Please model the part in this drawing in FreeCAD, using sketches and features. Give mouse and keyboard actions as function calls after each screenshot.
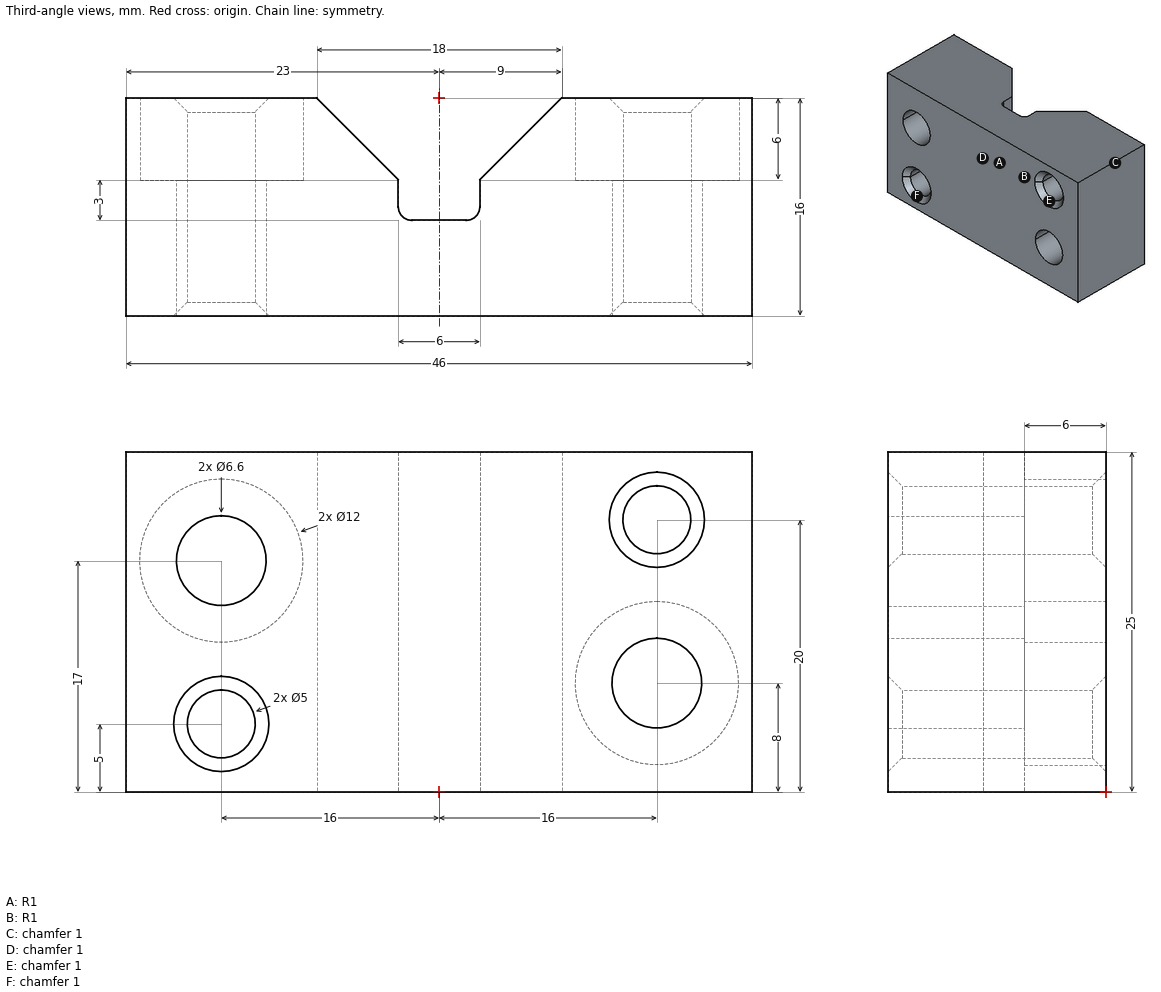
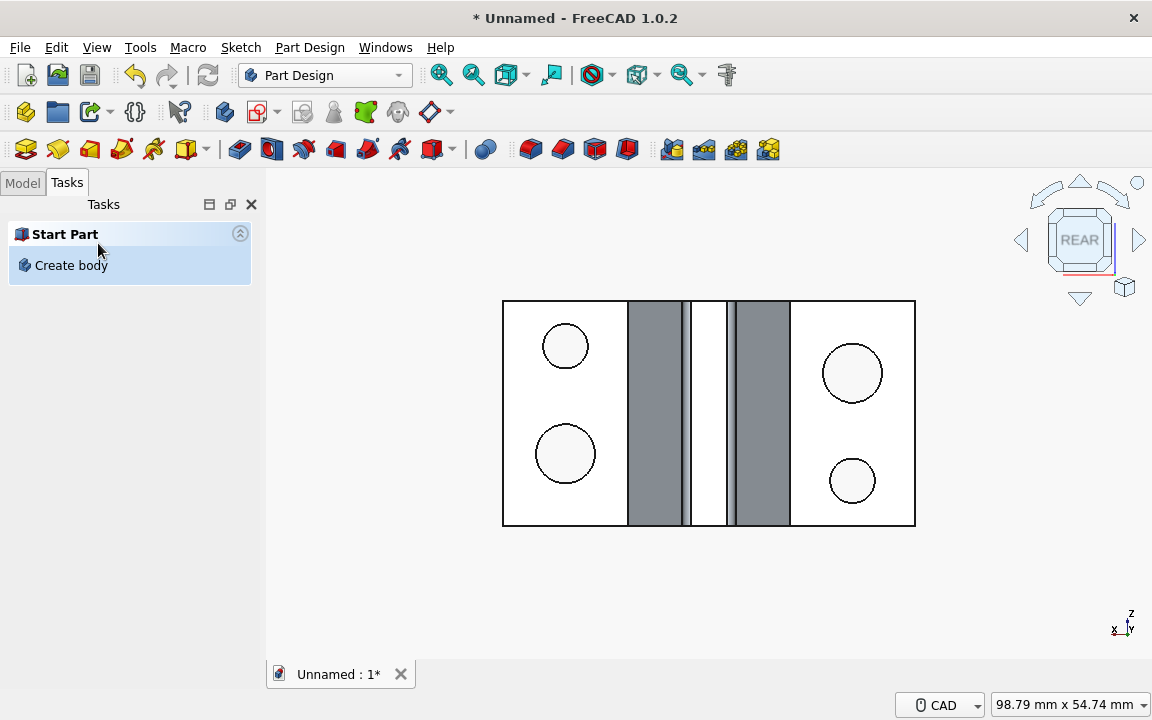
click(530, 380)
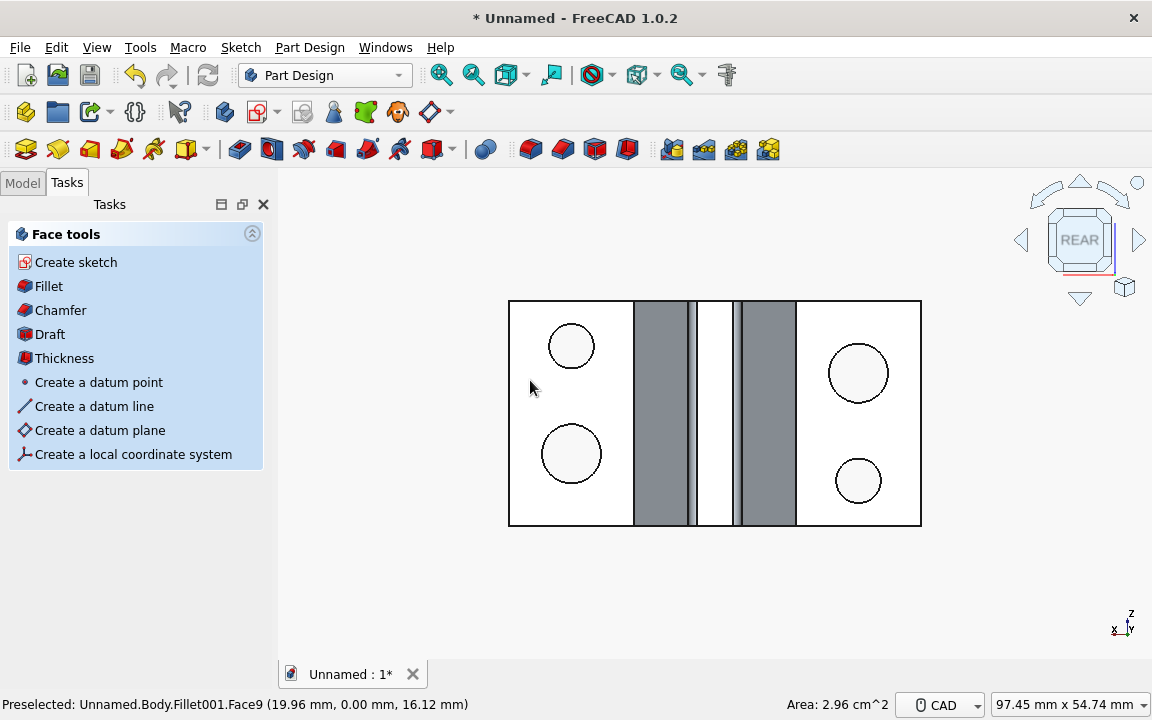
click(258, 112)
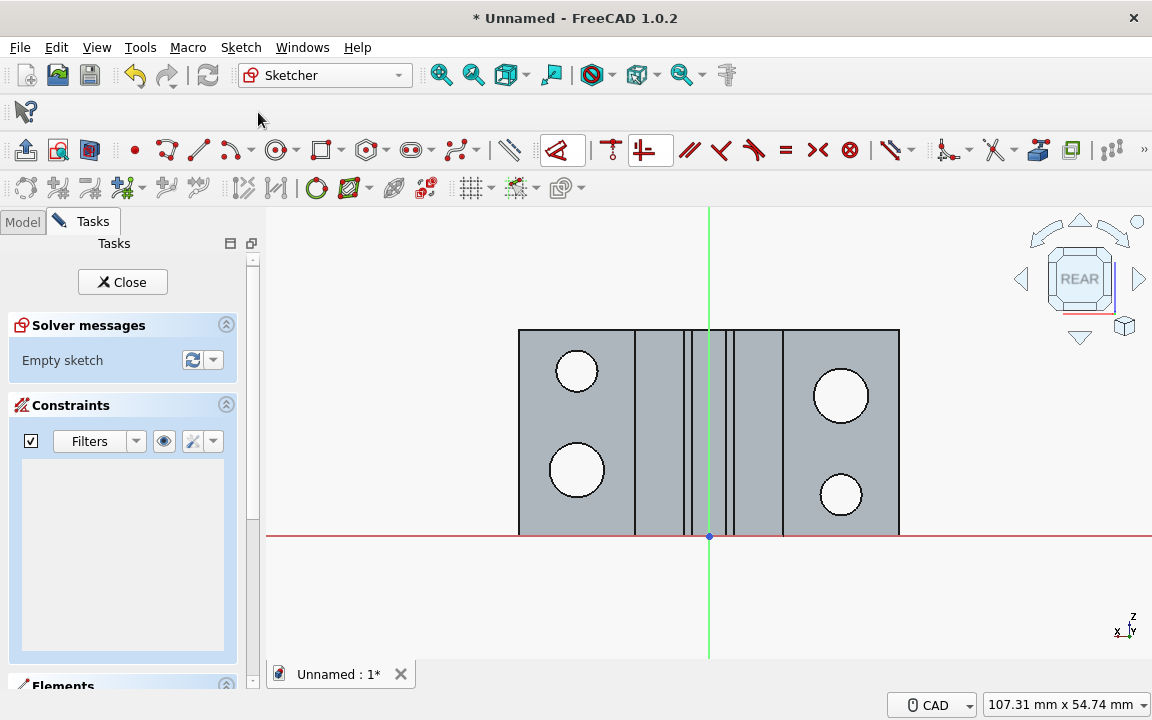
click(276, 150)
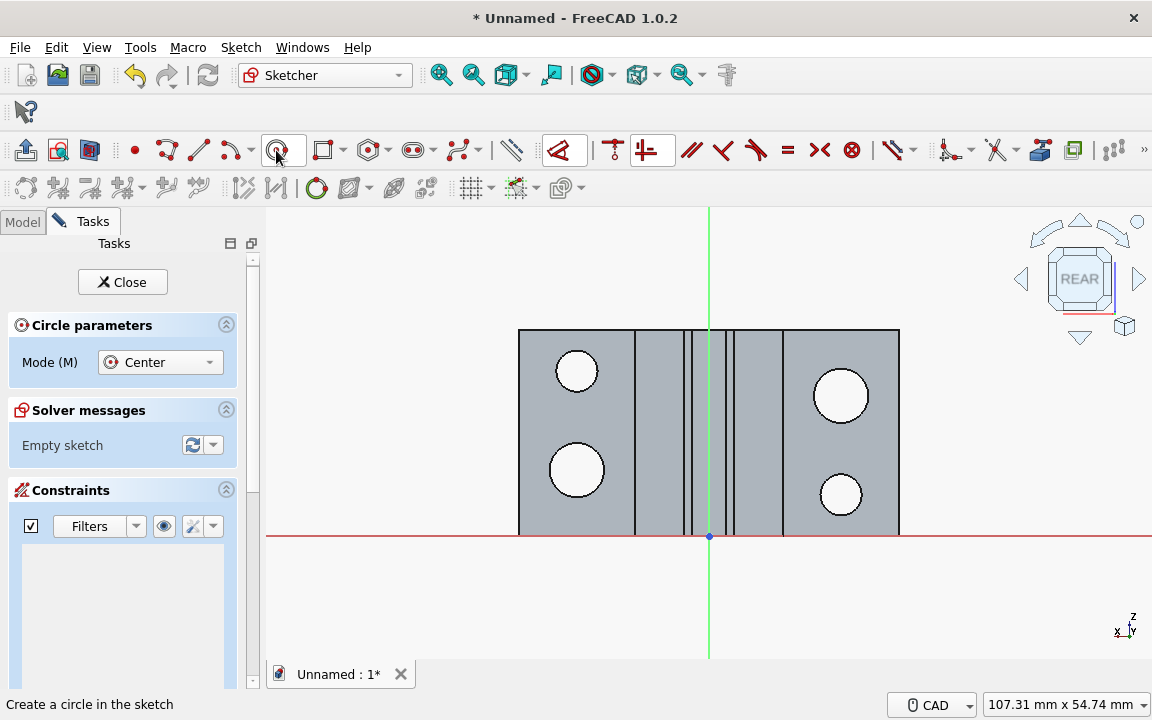
click(841, 396)
move(876, 361)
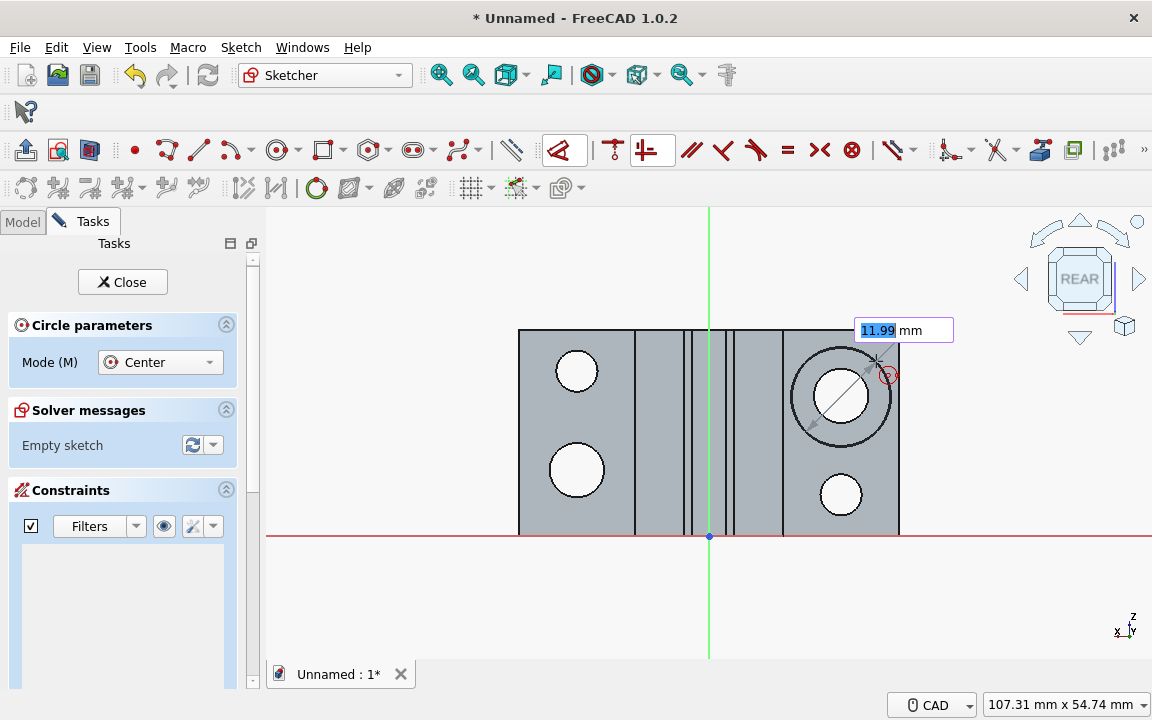
text(12)
key(Return)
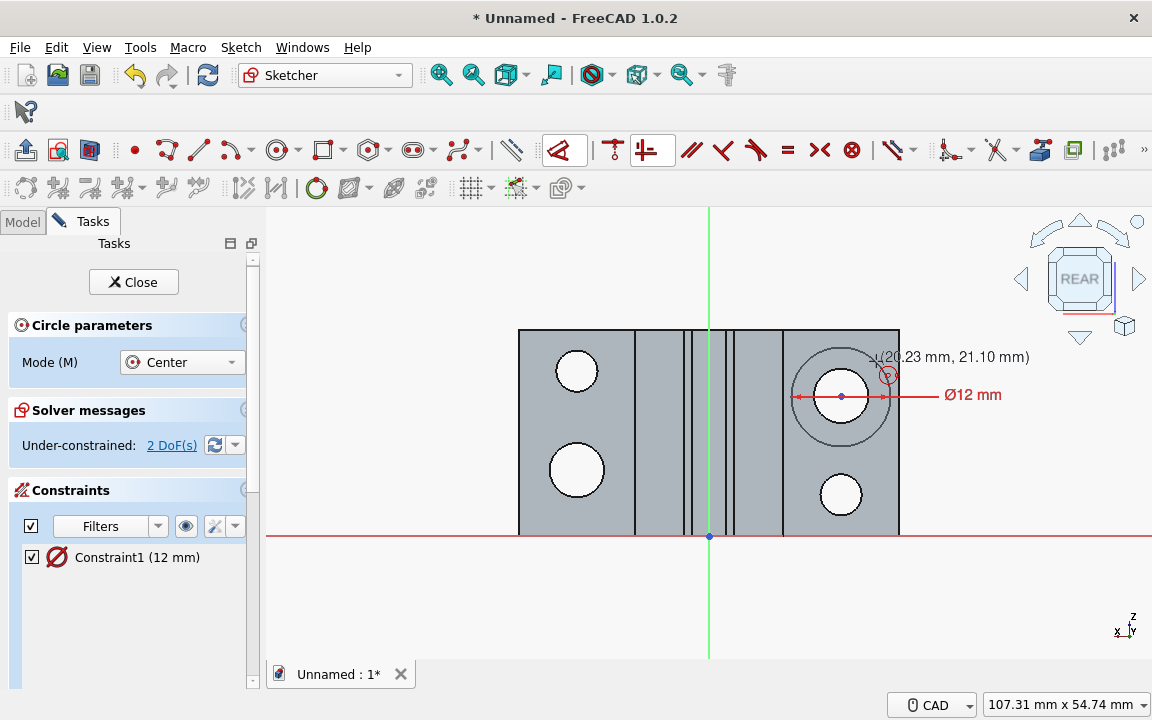
click(577, 470)
move(612, 435)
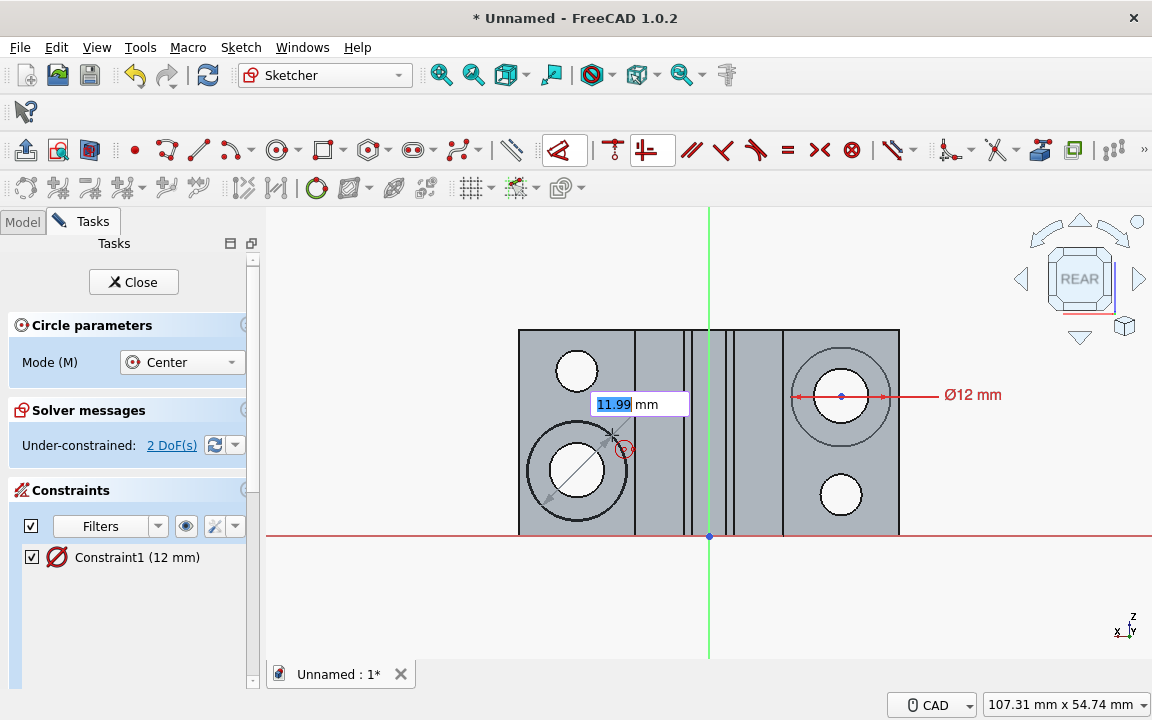
text(12)
key(Return)
key(Escape)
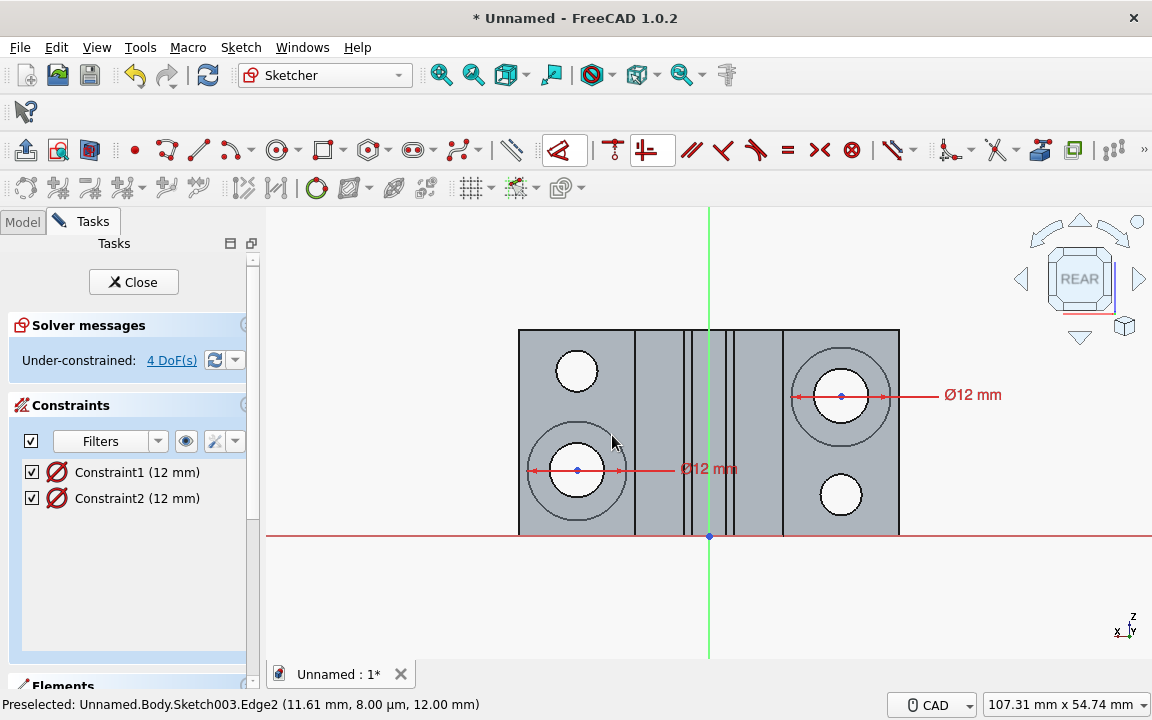
click(577, 471)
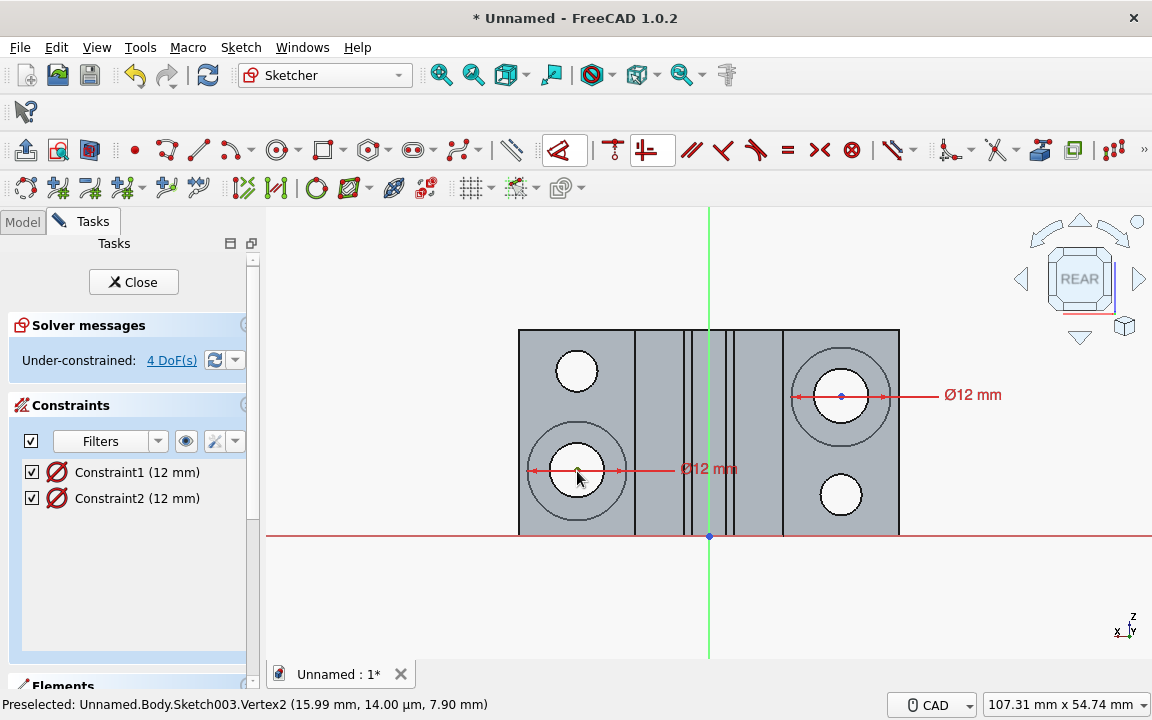
key(i)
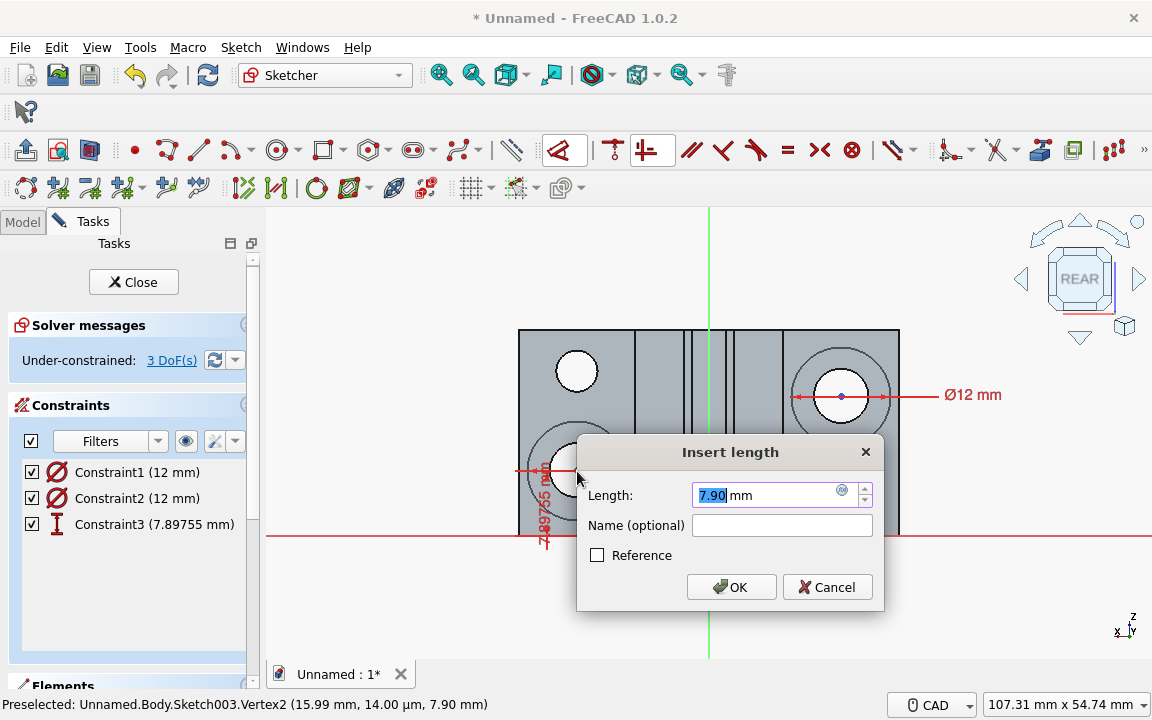
text(8)
key(Return)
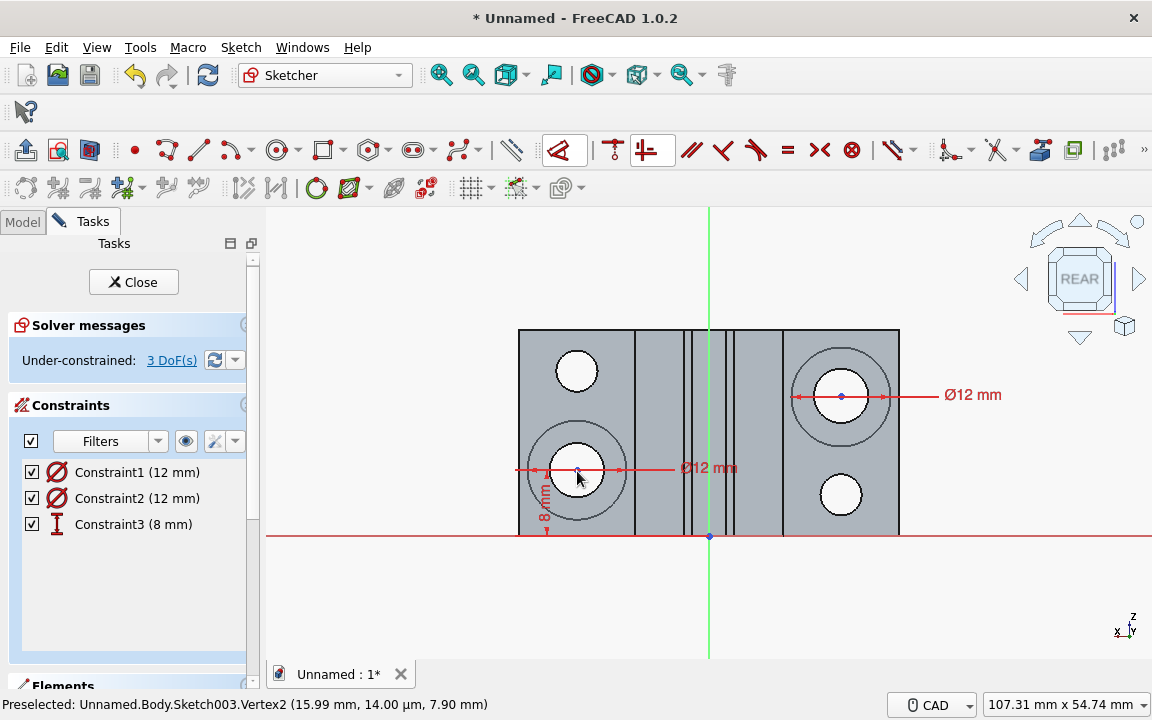
click(841, 397)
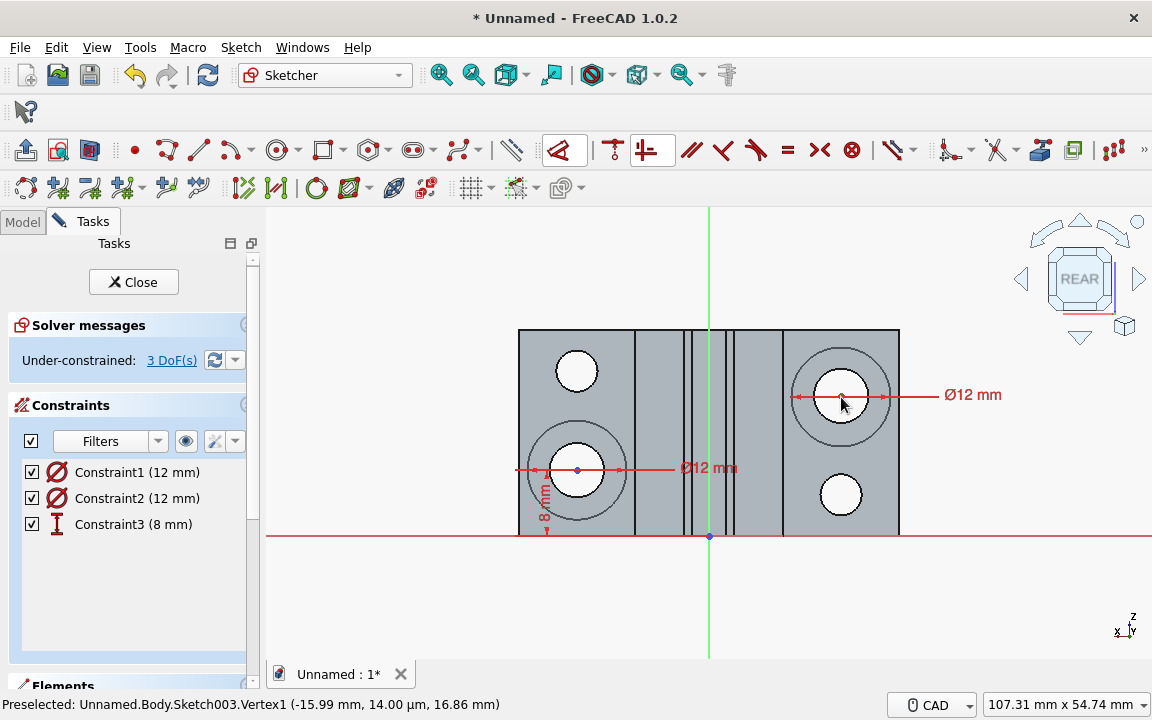
click(582, 150)